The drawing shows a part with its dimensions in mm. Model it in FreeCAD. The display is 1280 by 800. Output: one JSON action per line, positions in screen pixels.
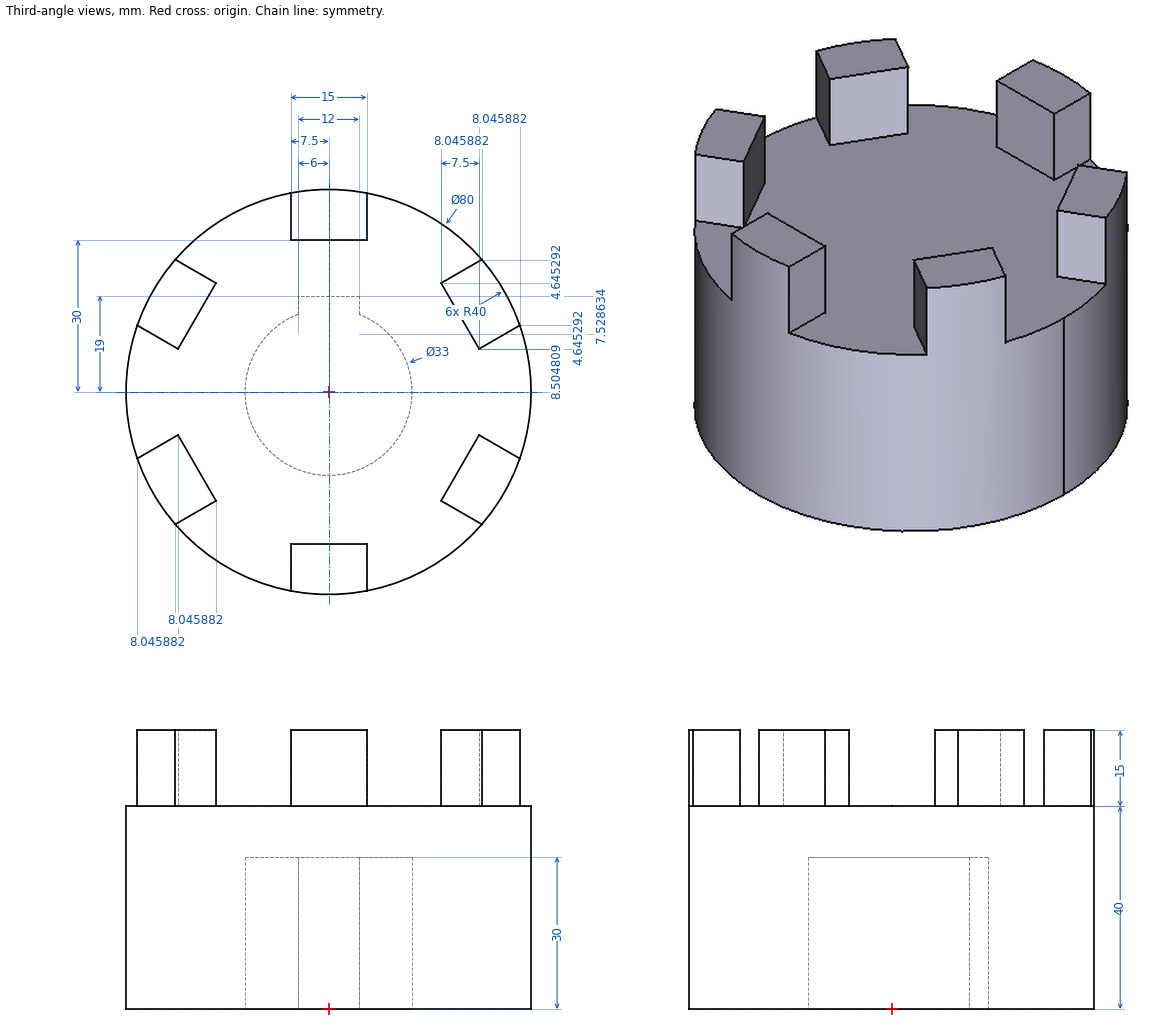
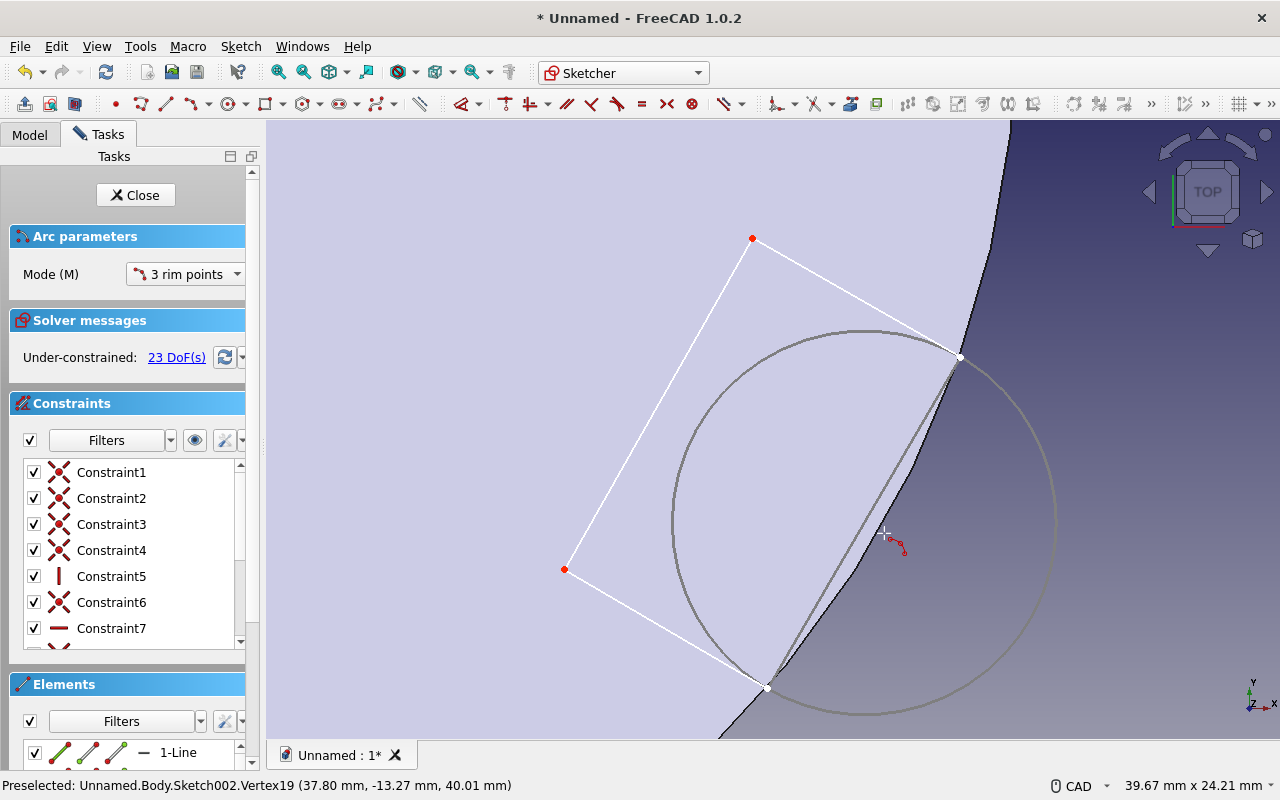
{"action": "left_click", "coordinate": [880, 529]}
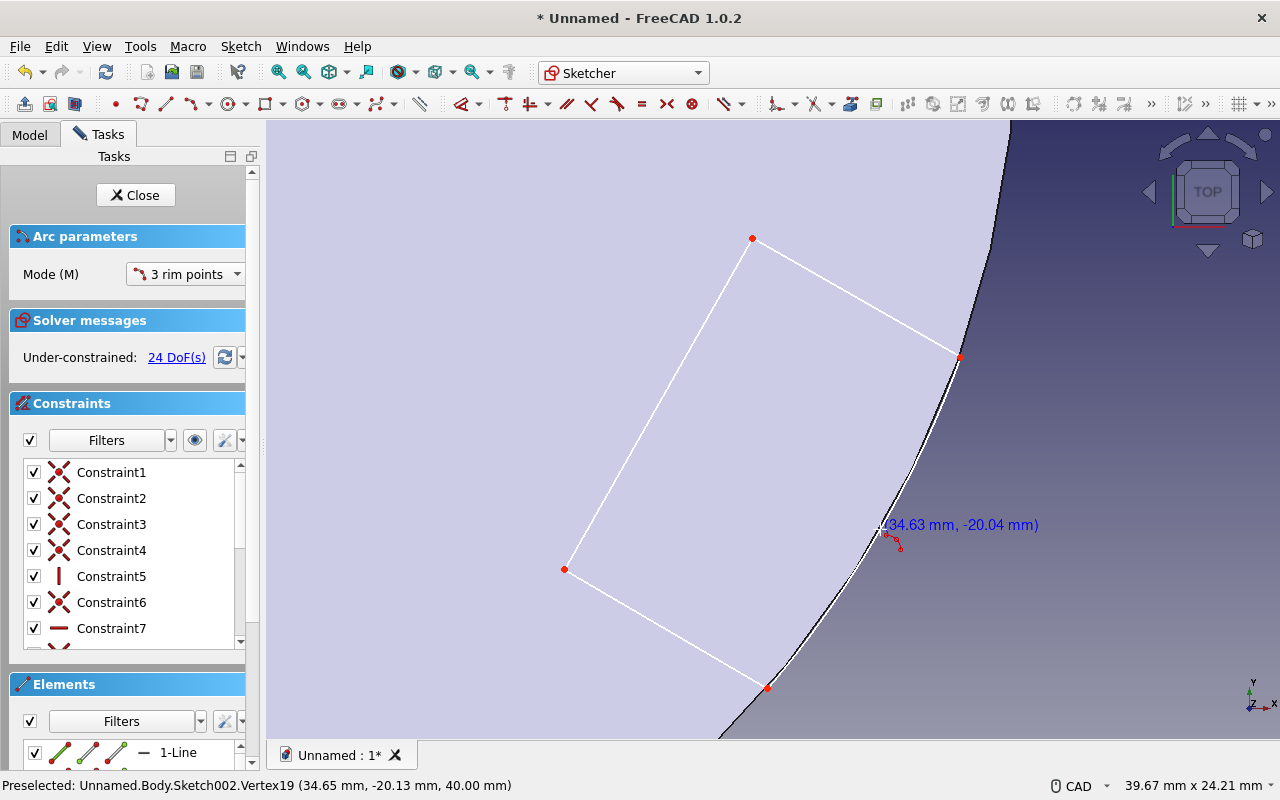
{"action": "key", "text": "g m"}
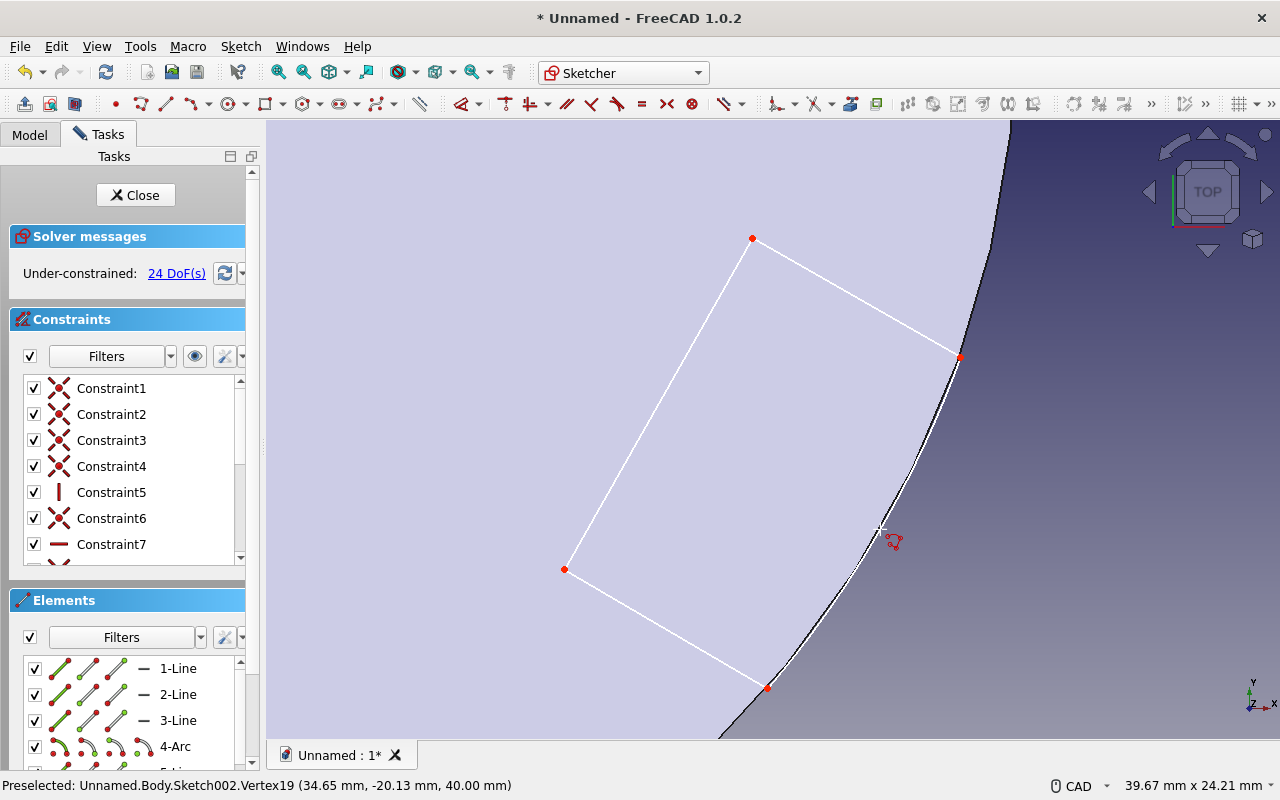
{"action": "scroll", "coordinate": [884, 534], "scroll_direction": "down", "scroll_amount": 8}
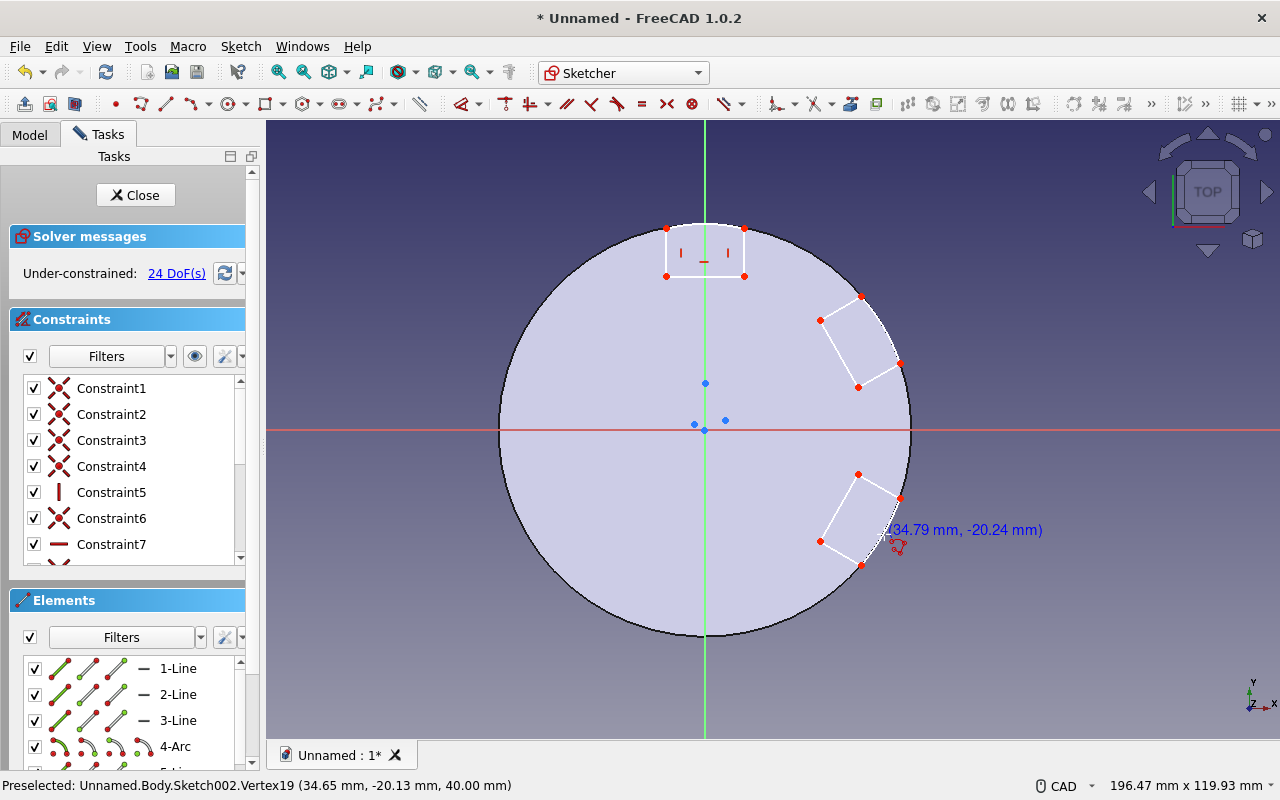
{"action": "left_click", "coordinate": [744, 633]}
{"action": "left_click", "coordinate": [744, 585]}
{"action": "left_click", "coordinate": [666, 585]}
{"action": "left_click", "coordinate": [666, 633]}
{"action": "right_click", "coordinate": [666, 633]}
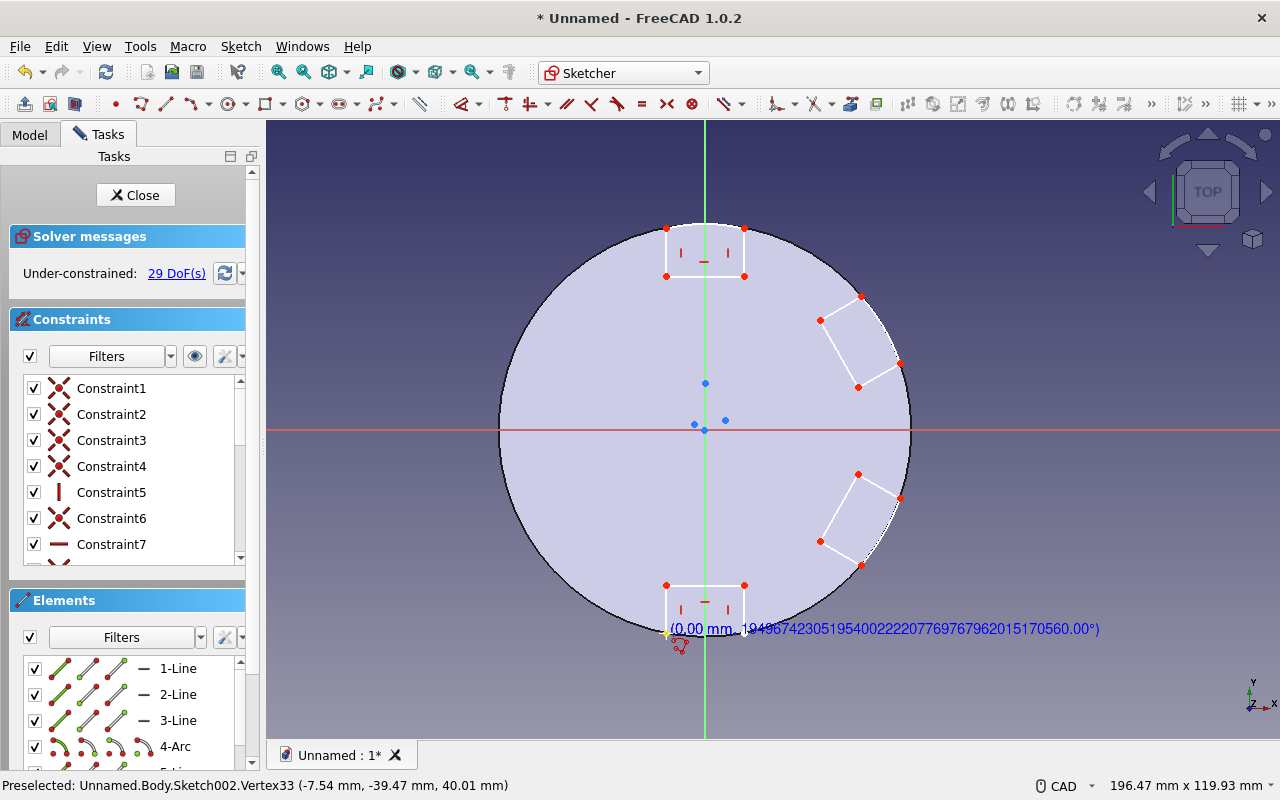
{"action": "key", "text": "g 3 a"}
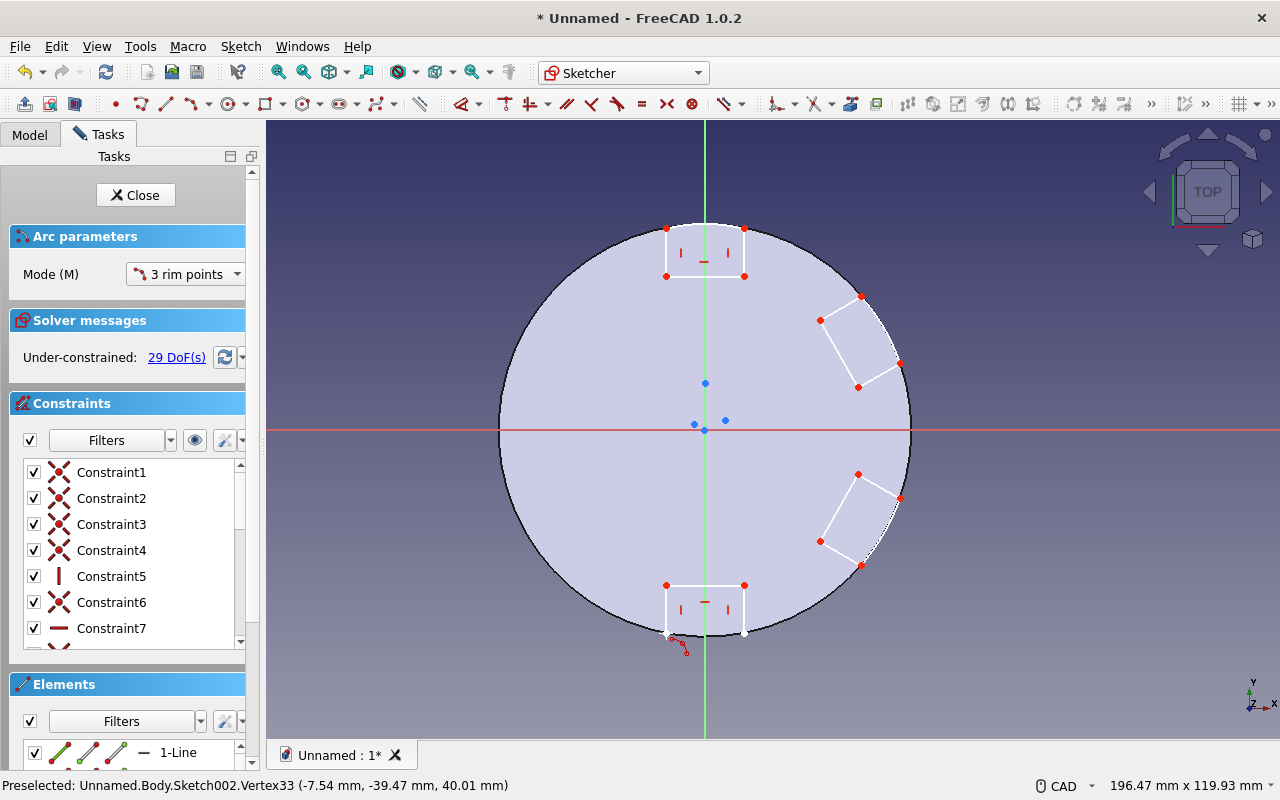
{"action": "left_click", "coordinate": [666, 634]}
{"action": "left_click", "coordinate": [744, 634]}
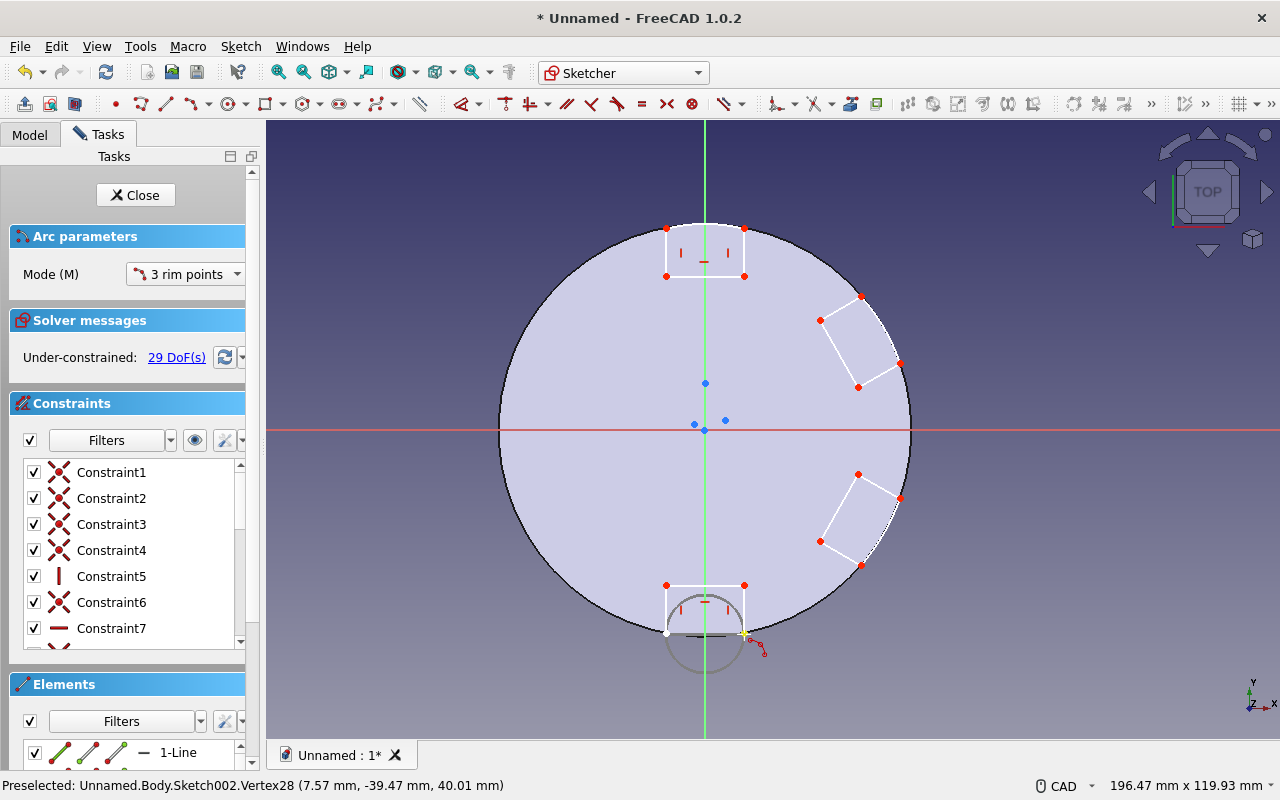
{"action": "scroll", "coordinate": [697, 637], "scroll_direction": "up", "scroll_amount": 8}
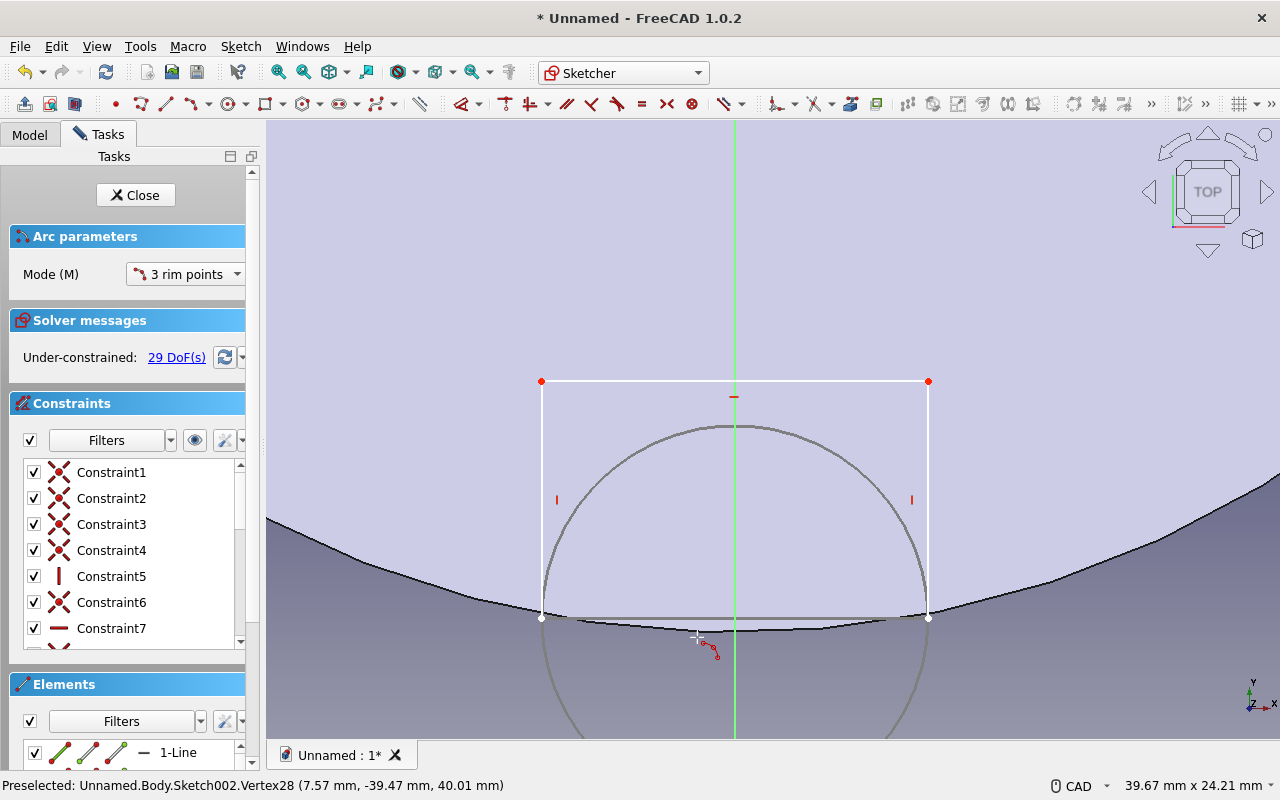
{"action": "left_click", "coordinate": [696, 632]}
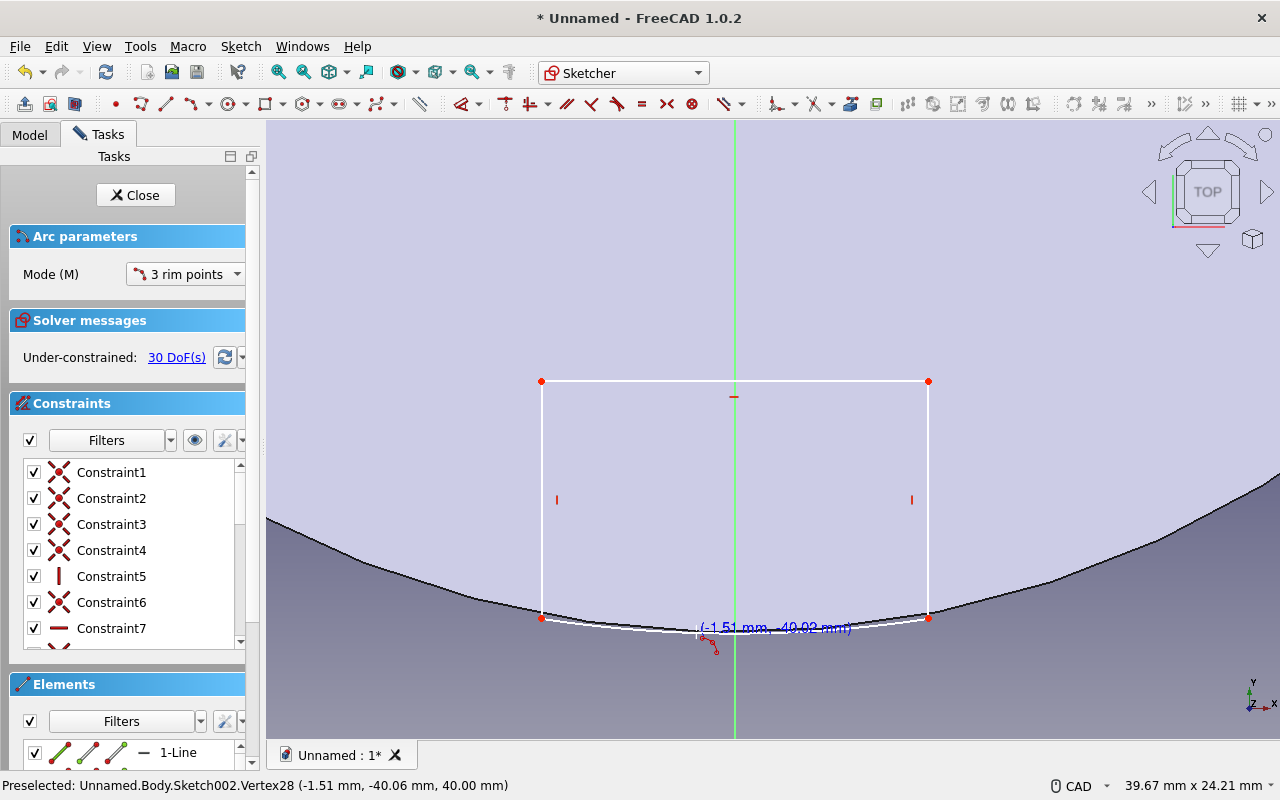
{"action": "left_click", "coordinate": [141, 104]}